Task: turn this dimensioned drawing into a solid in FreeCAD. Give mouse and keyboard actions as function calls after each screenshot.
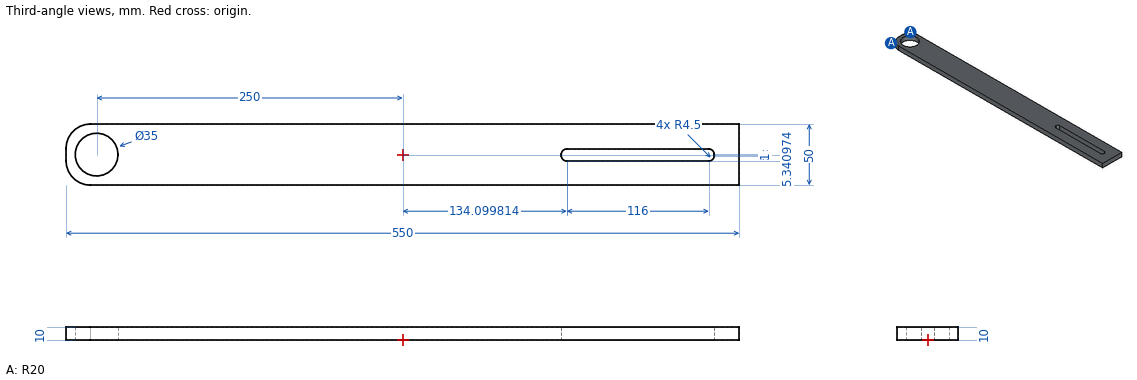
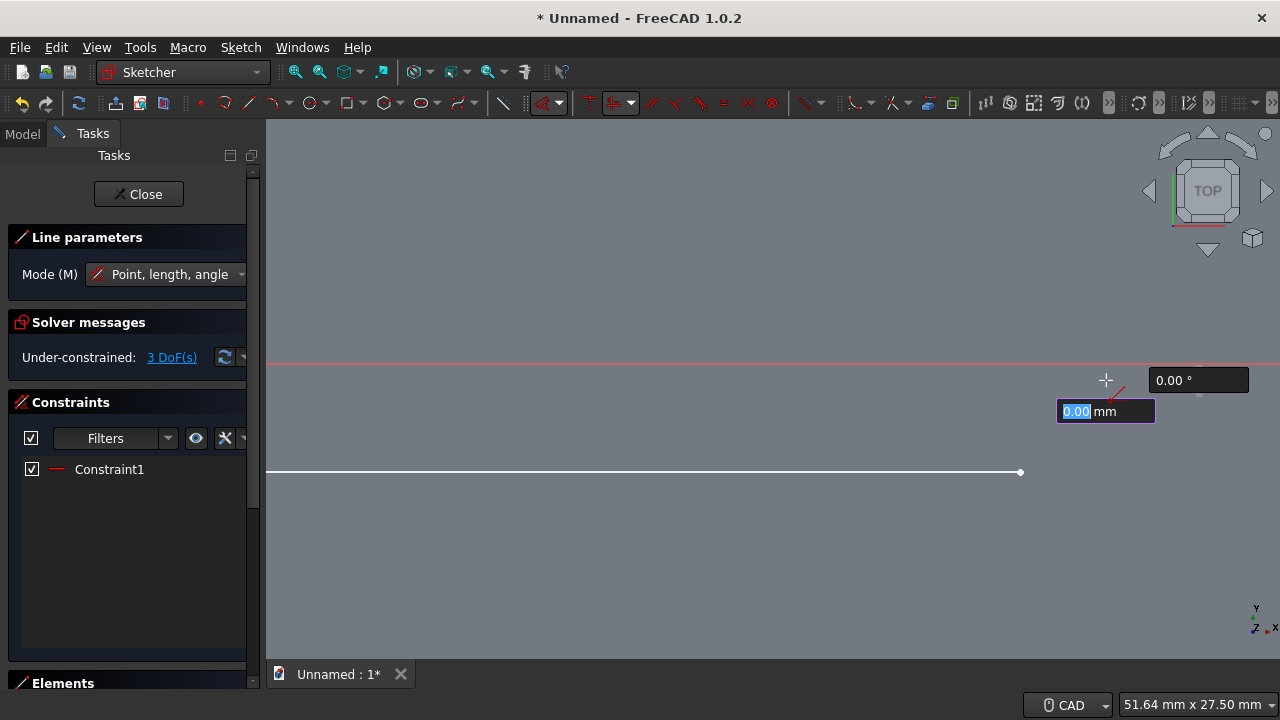
scroll(1106, 361, up, 9)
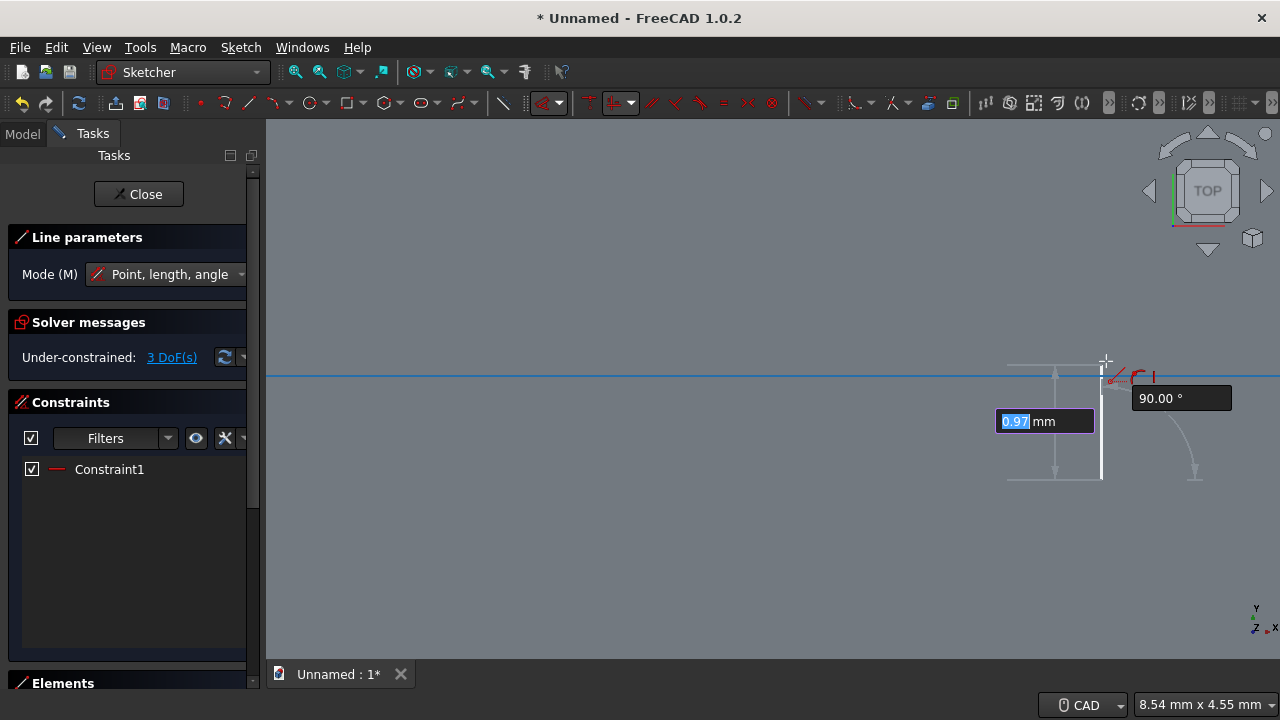
click(1102, 357)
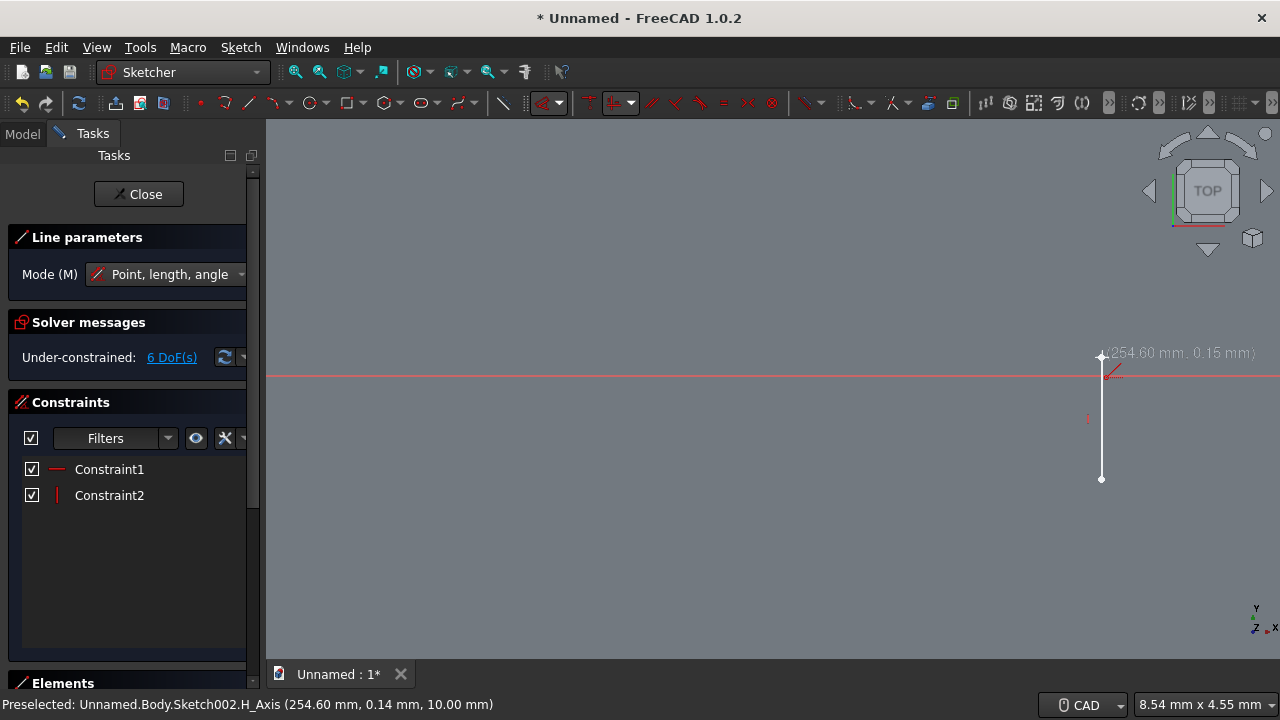
scroll(704, 389, down, 15)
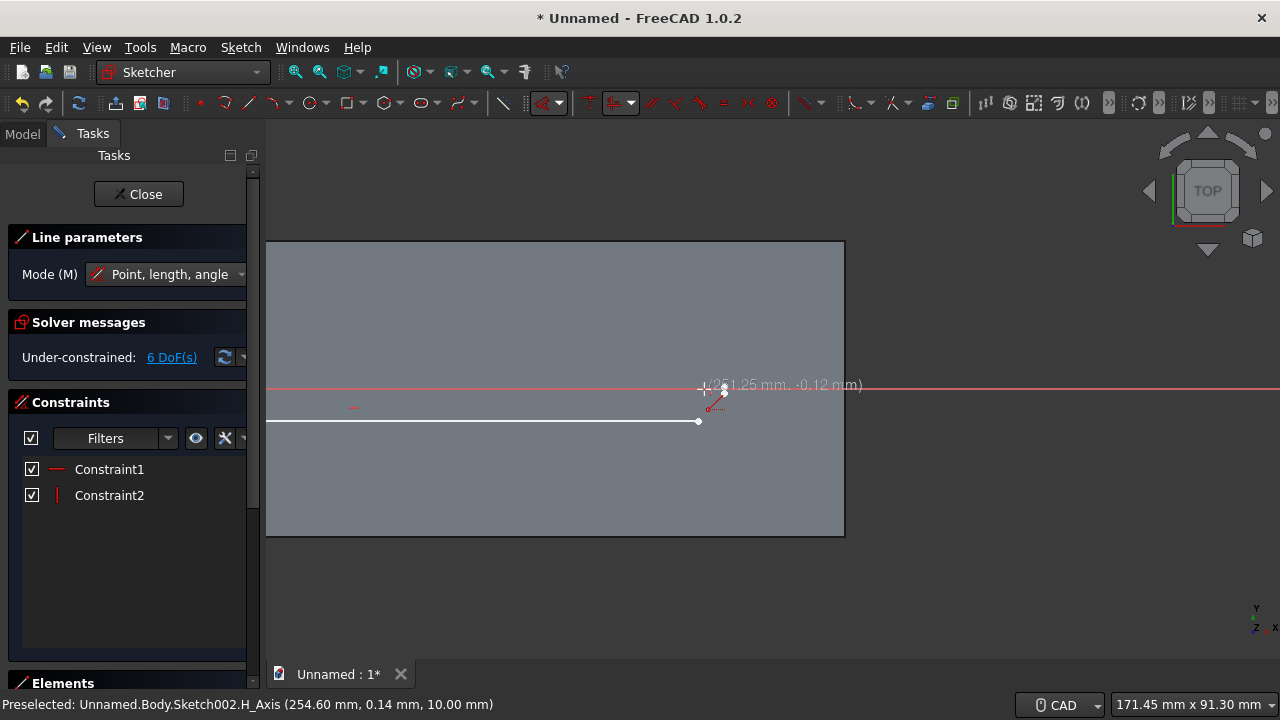
scroll(1115, 388, down, 5)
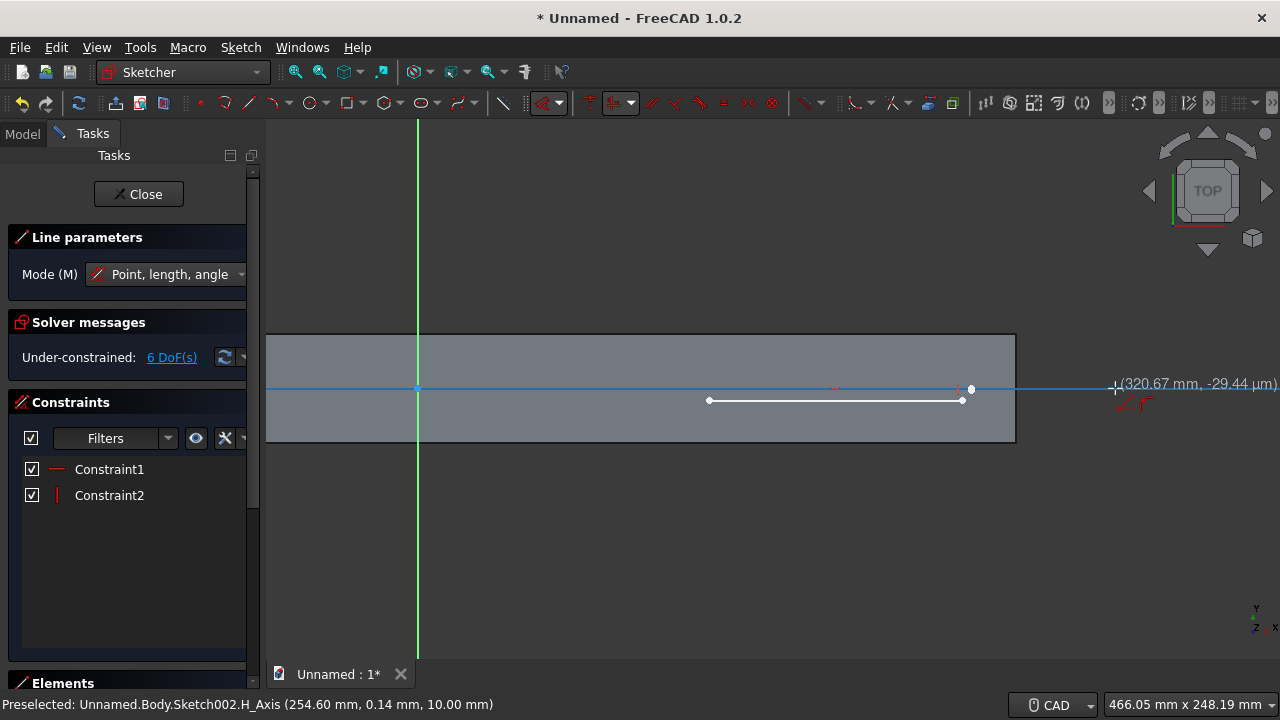
scroll(962, 378, up, 3)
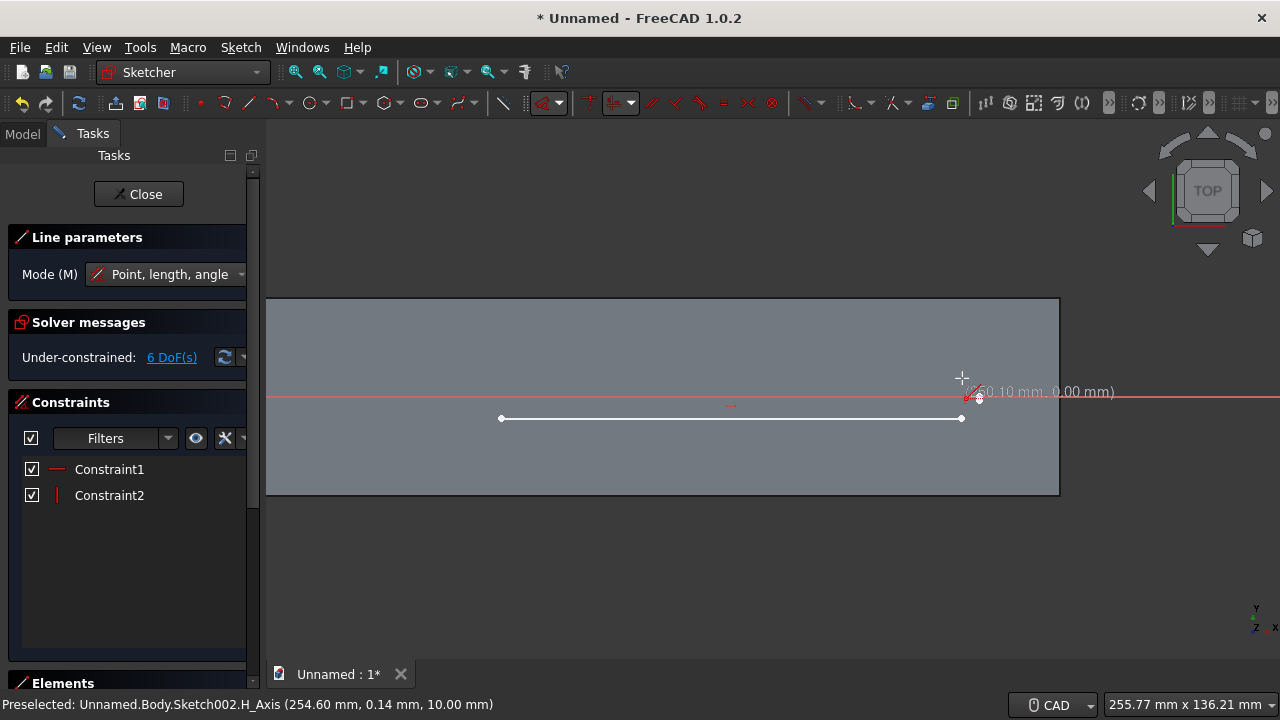
click(961, 378)
click(502, 378)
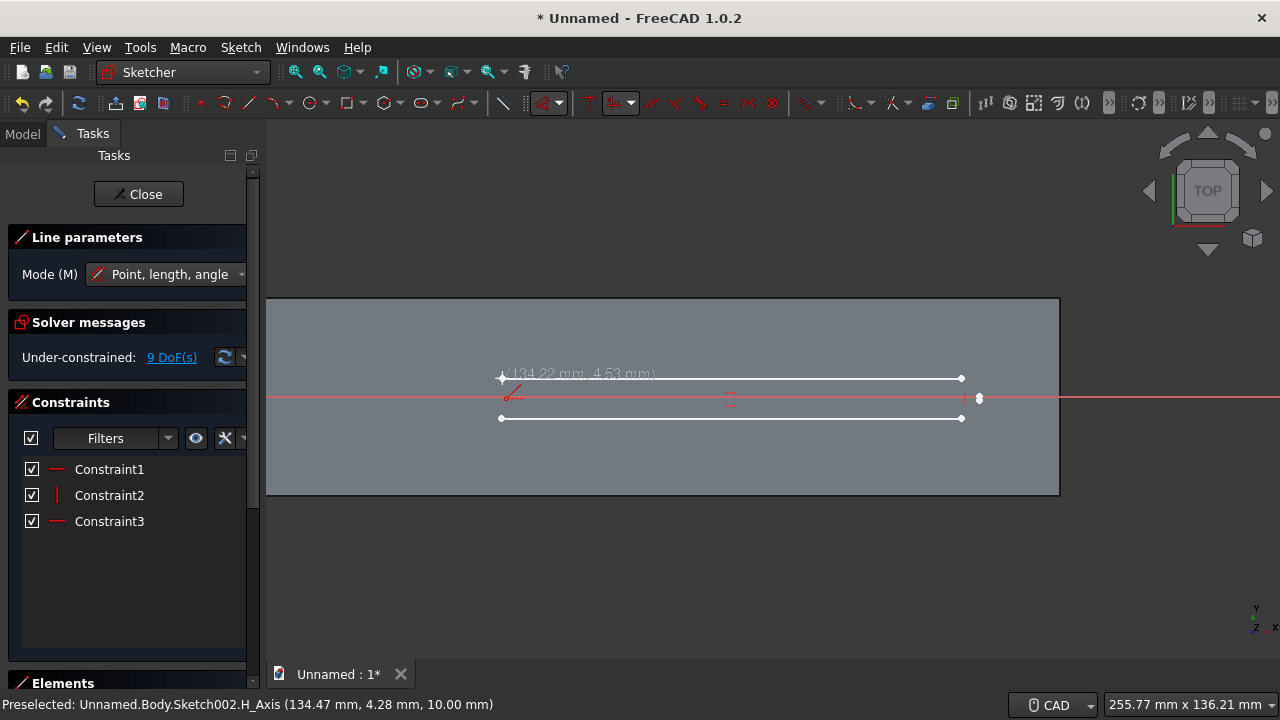
scroll(484, 396, up, 17)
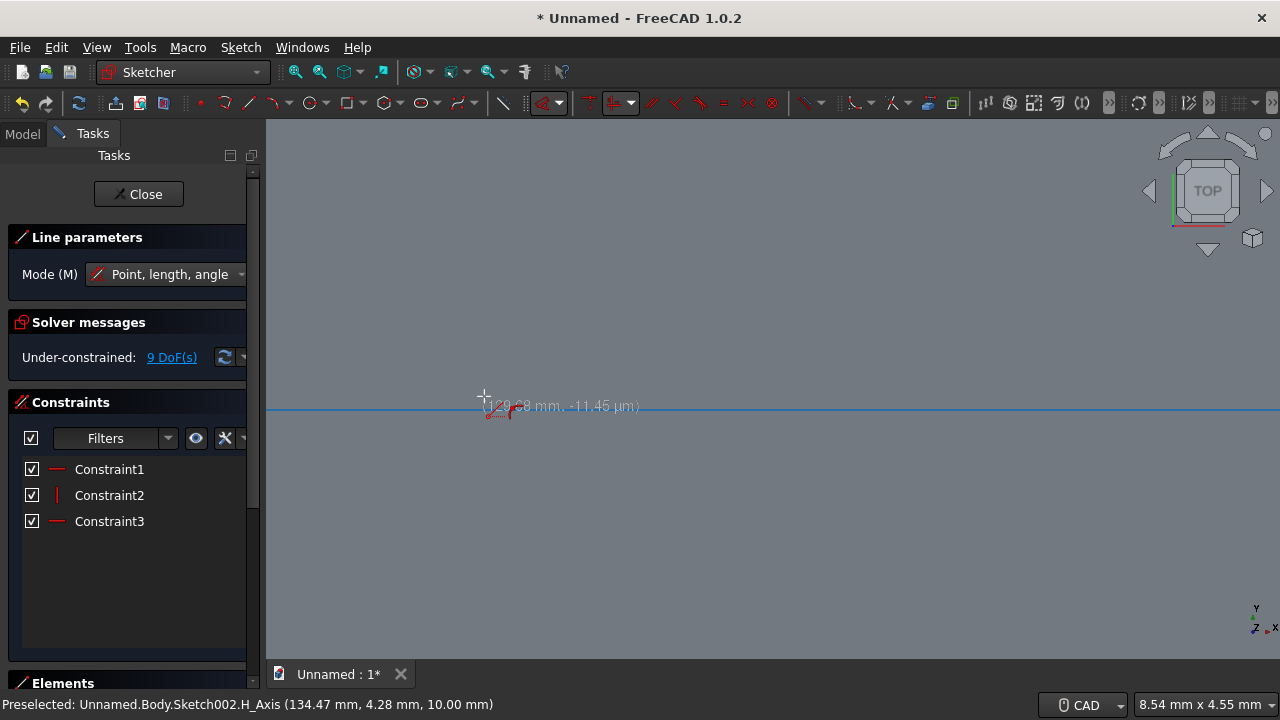
click(469, 391)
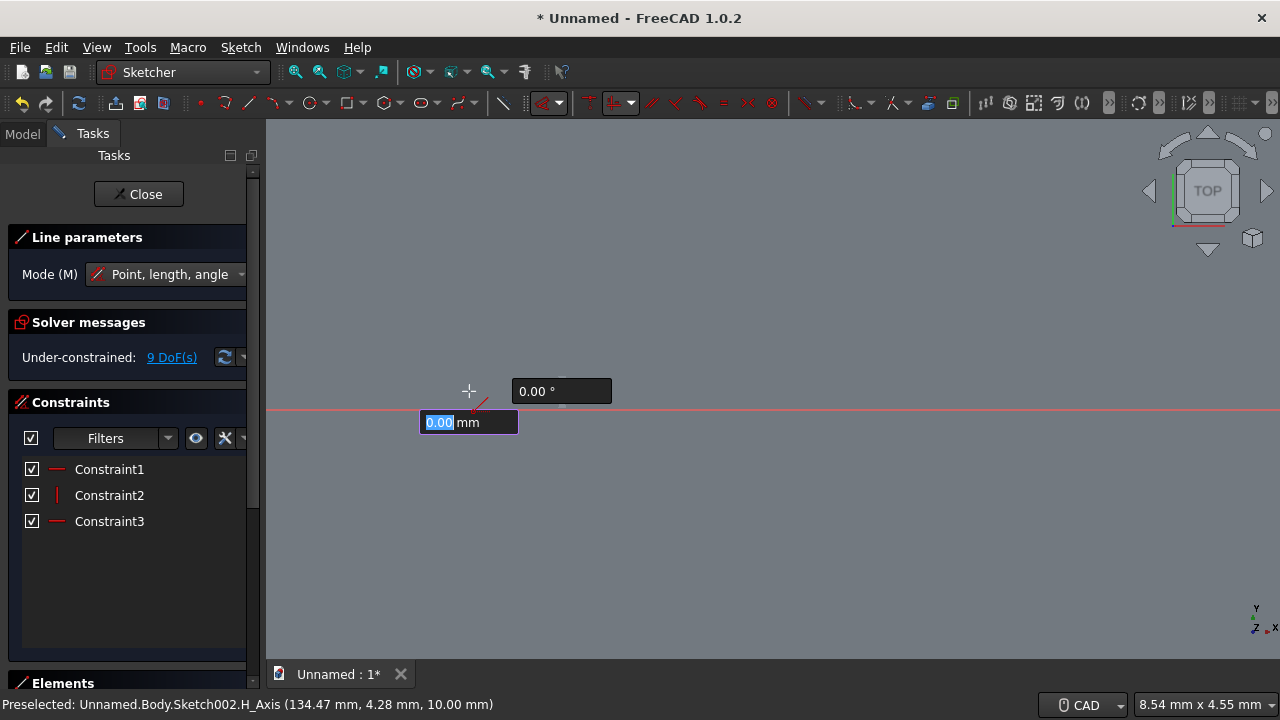
scroll(704, 389, down, 15)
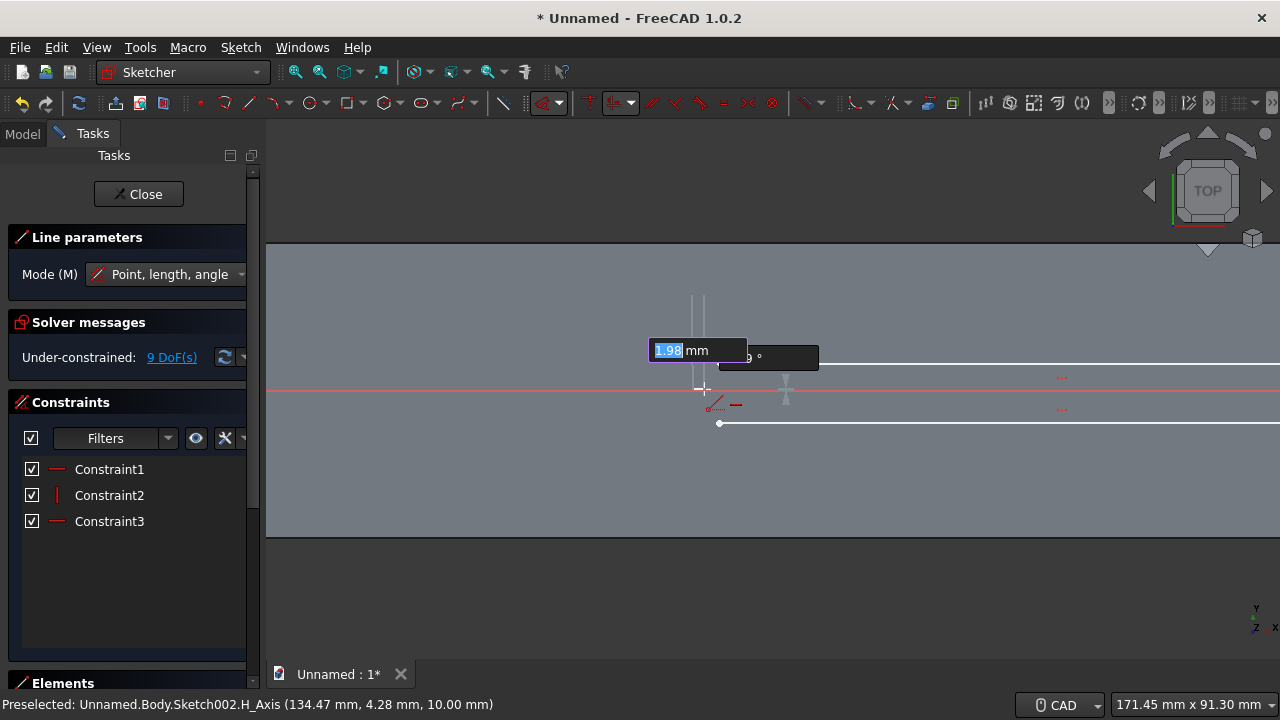
scroll(719, 387, down, 5)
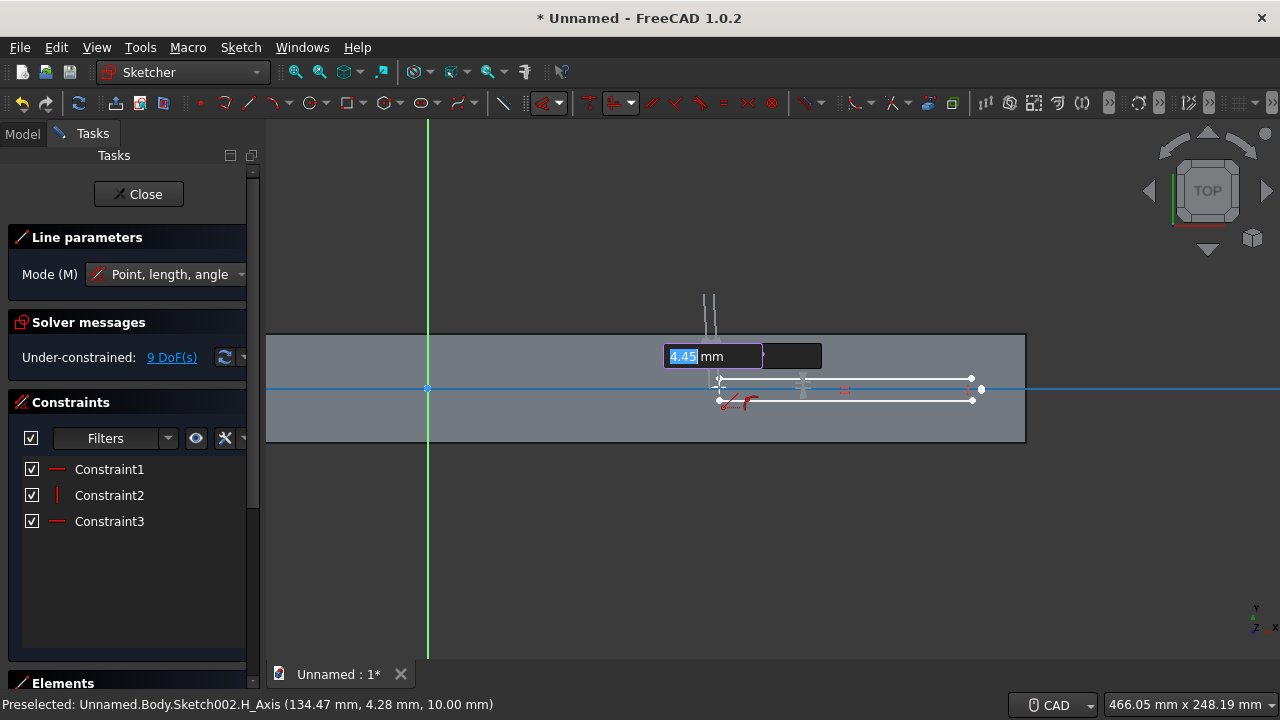
scroll(710, 390, up, 11)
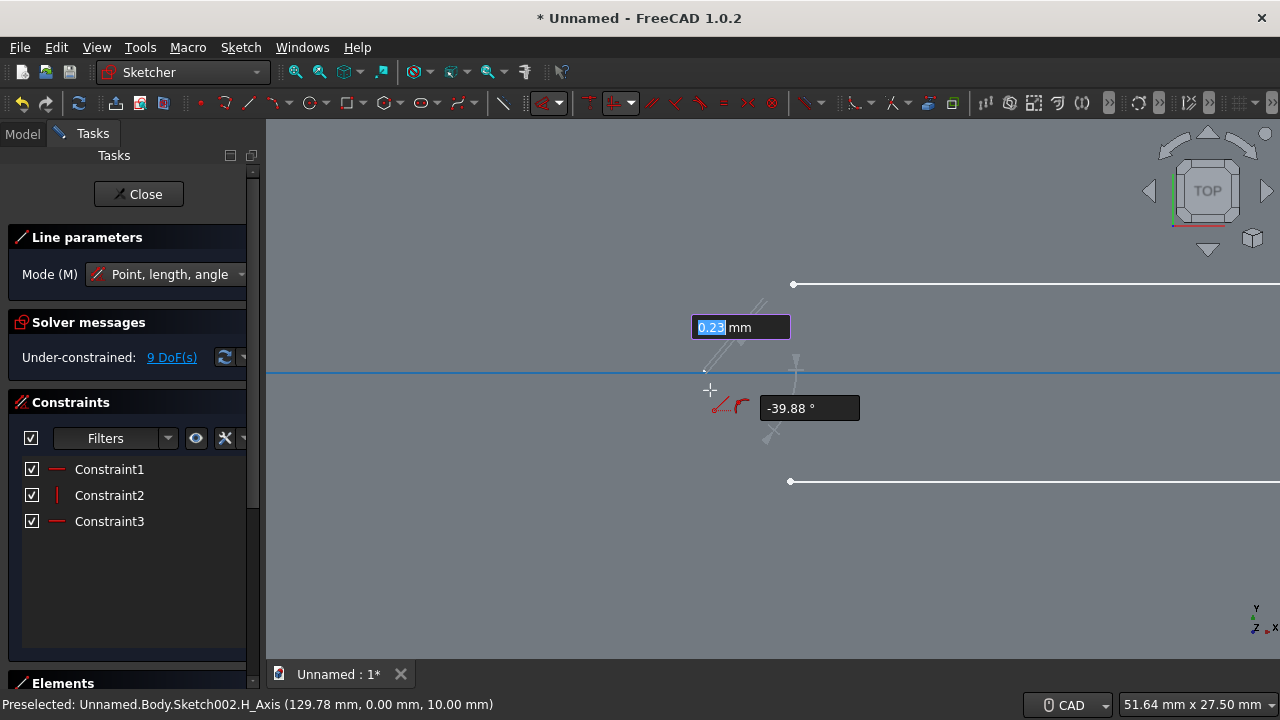
click(703, 390)